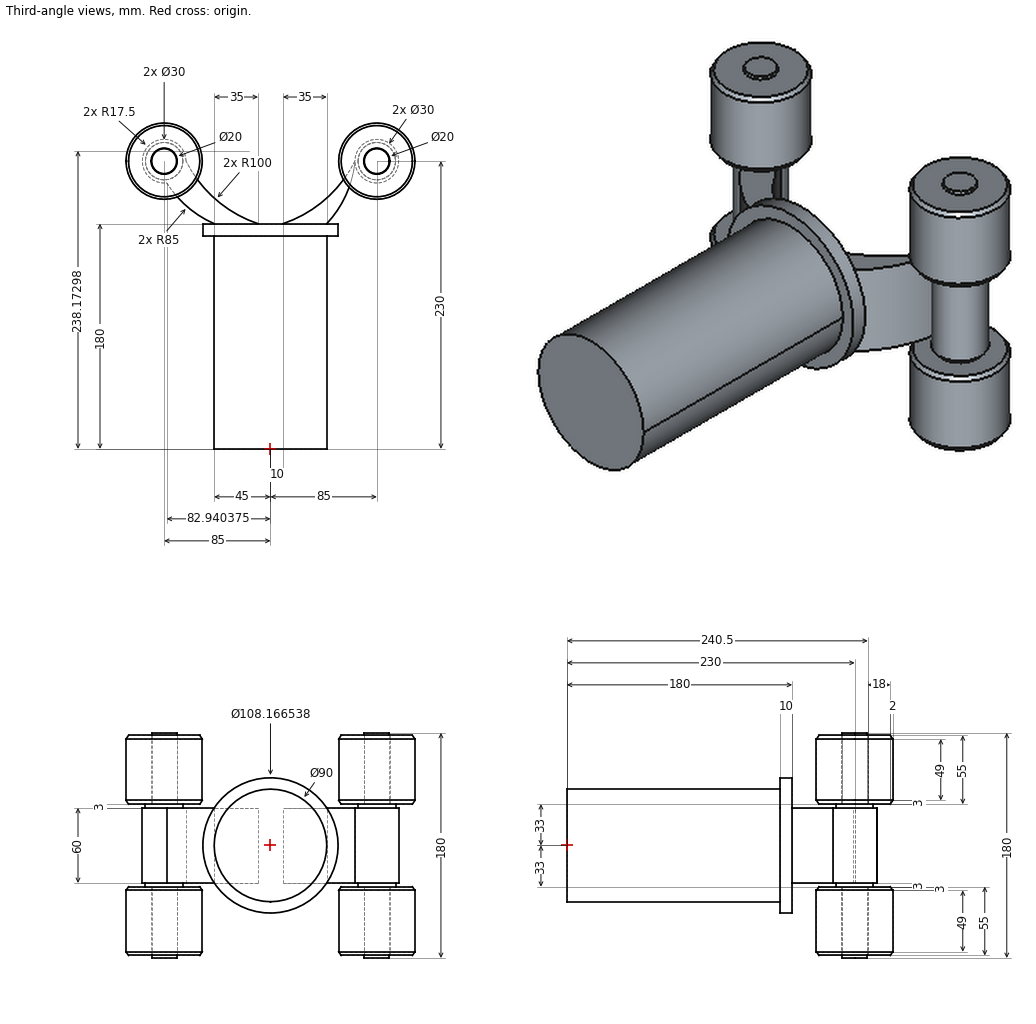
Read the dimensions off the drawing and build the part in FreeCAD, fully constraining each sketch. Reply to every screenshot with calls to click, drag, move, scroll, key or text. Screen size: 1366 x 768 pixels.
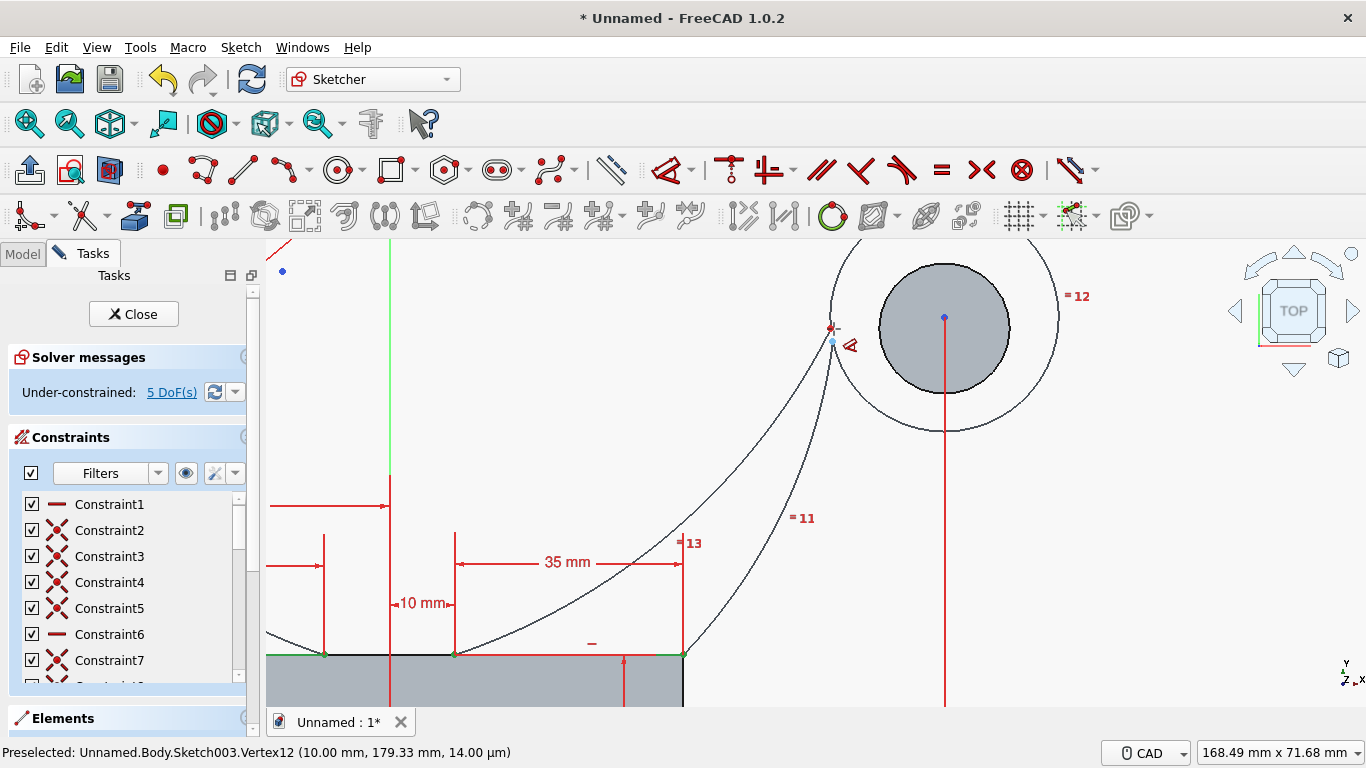
click(831, 329)
click(865, 504)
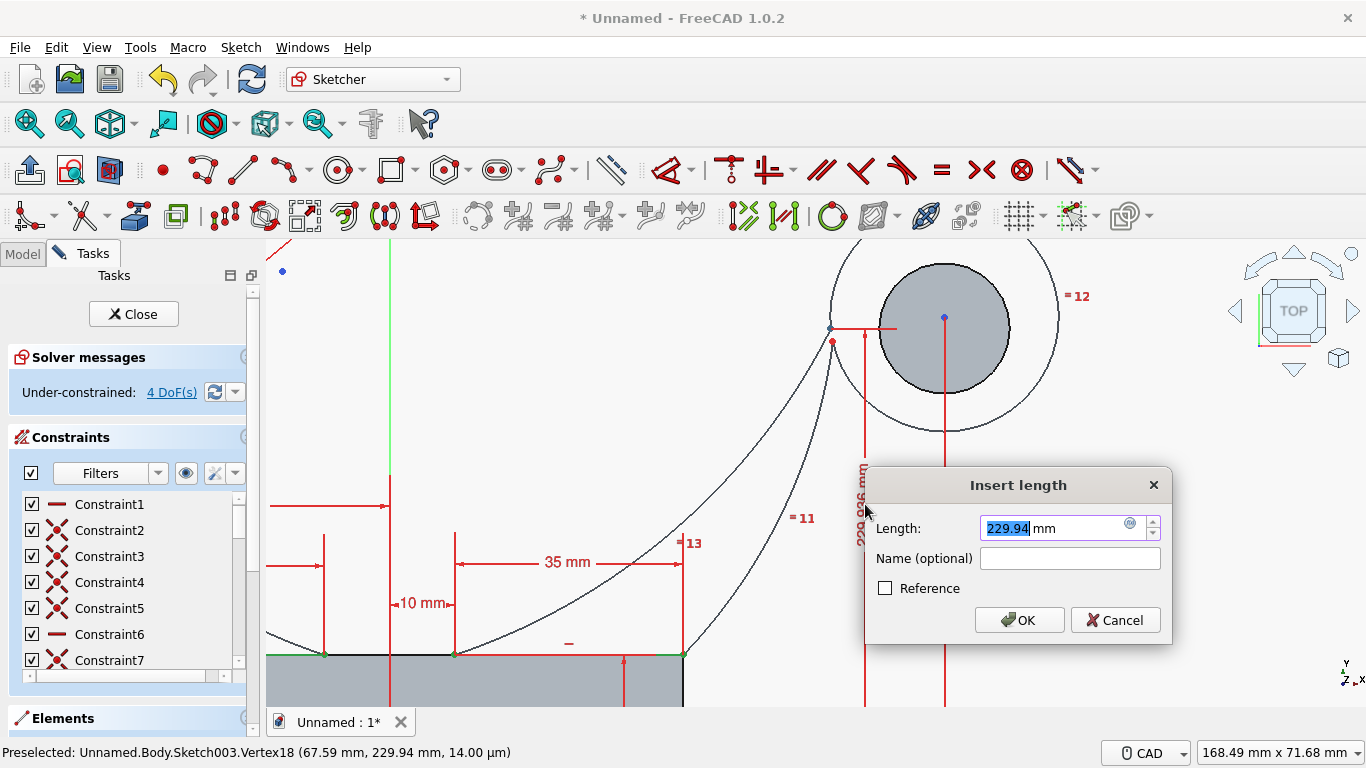
text(230)
key(Return)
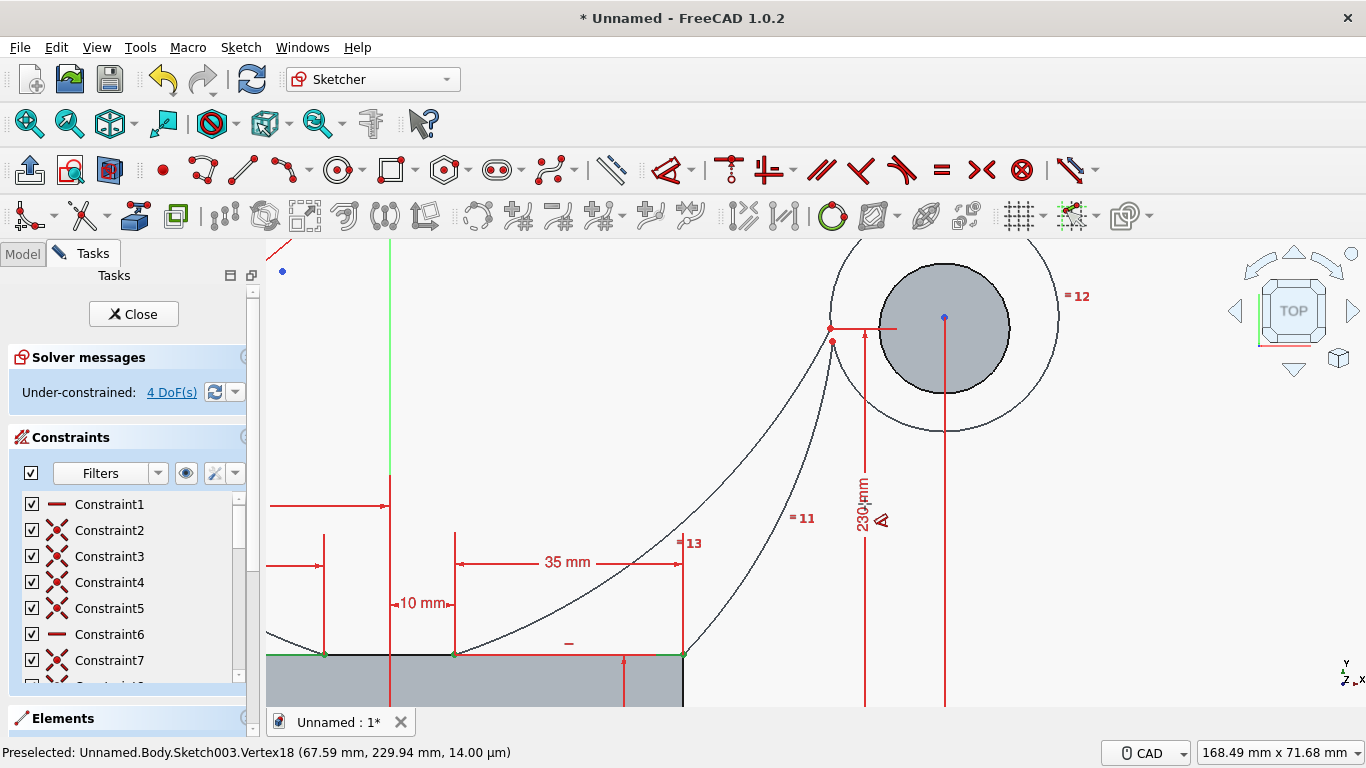
scroll(834, 329, down, 8)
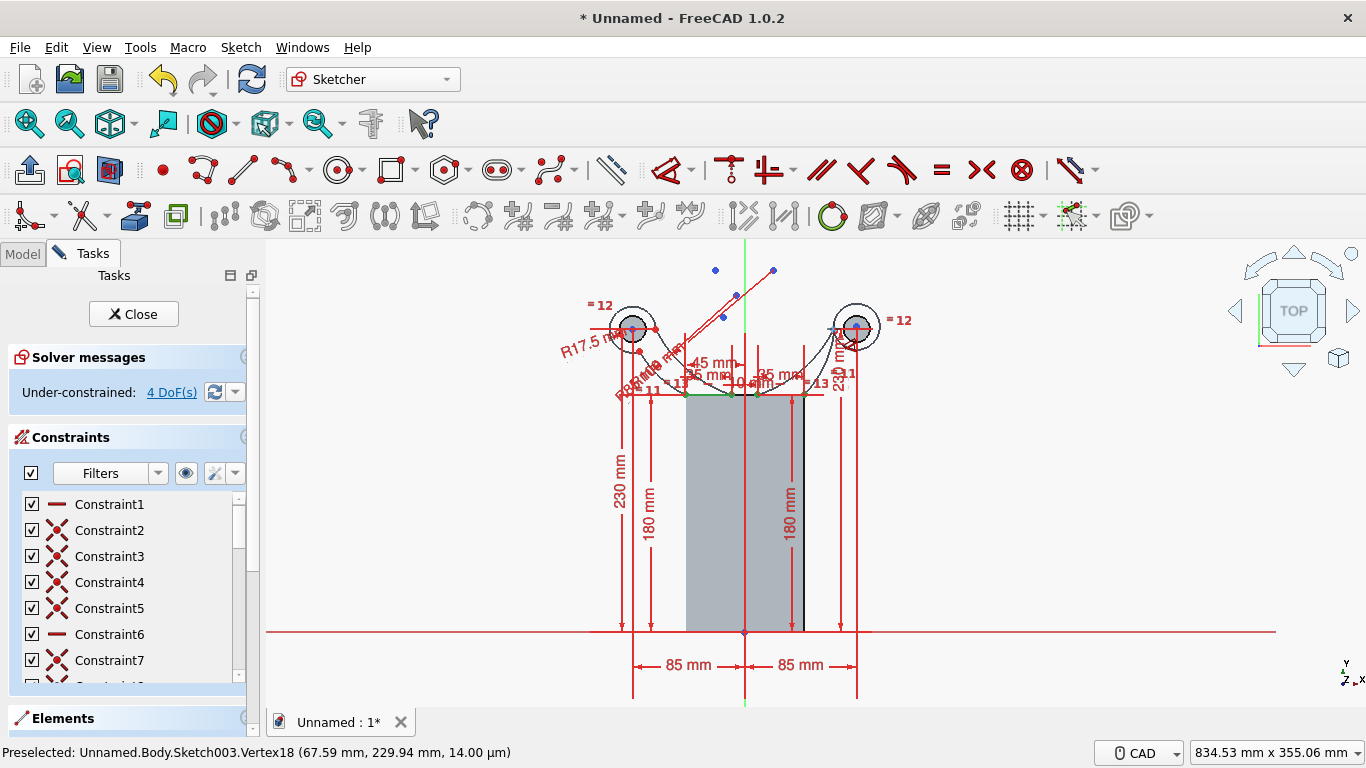
click(633, 330)
click(599, 411)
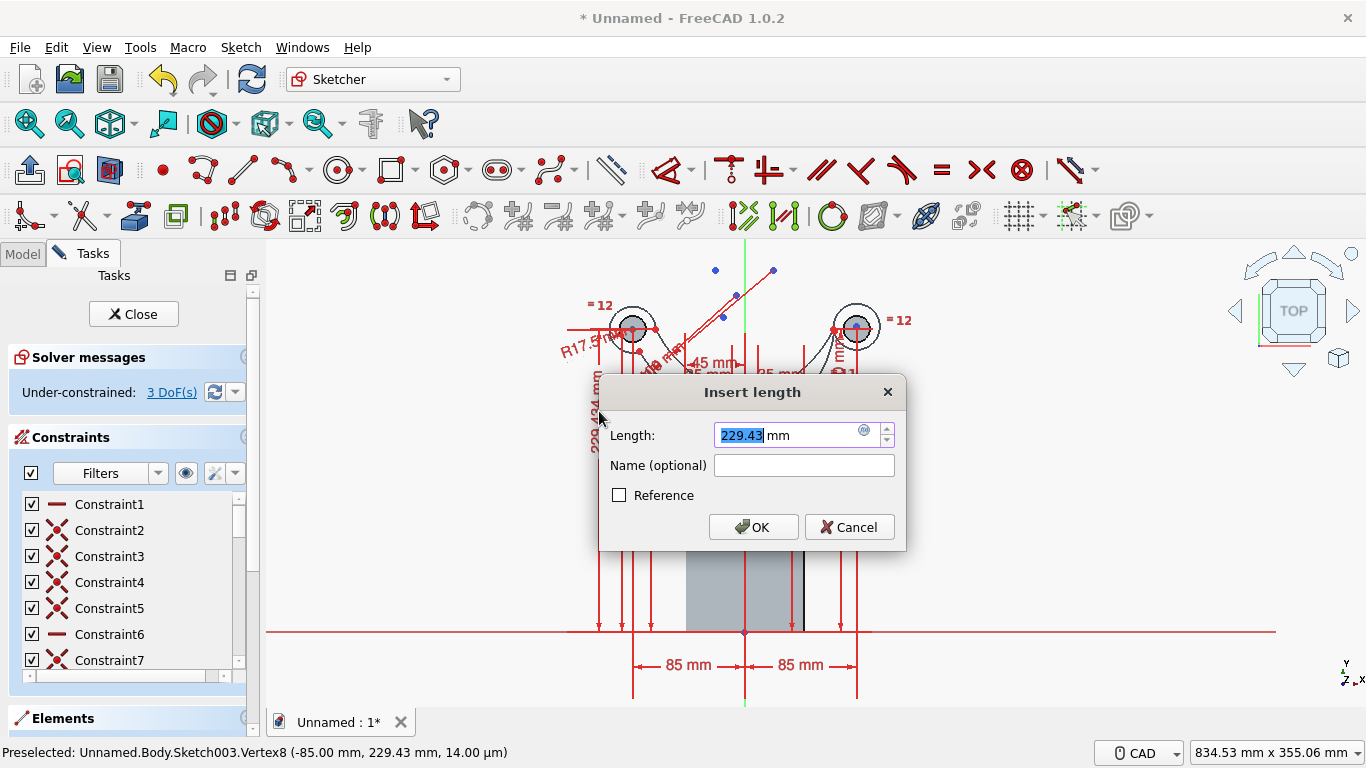
text(230)
key(Return)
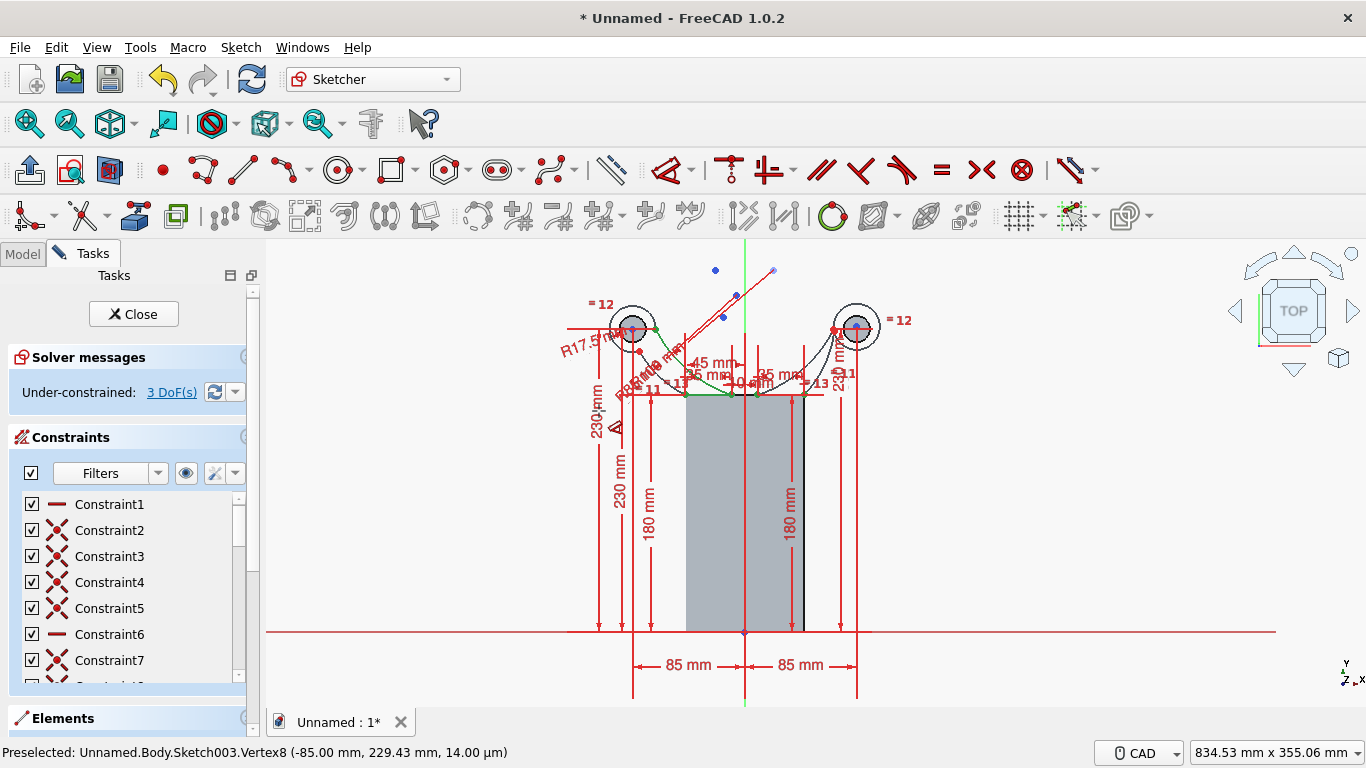
click(857, 327)
click(891, 480)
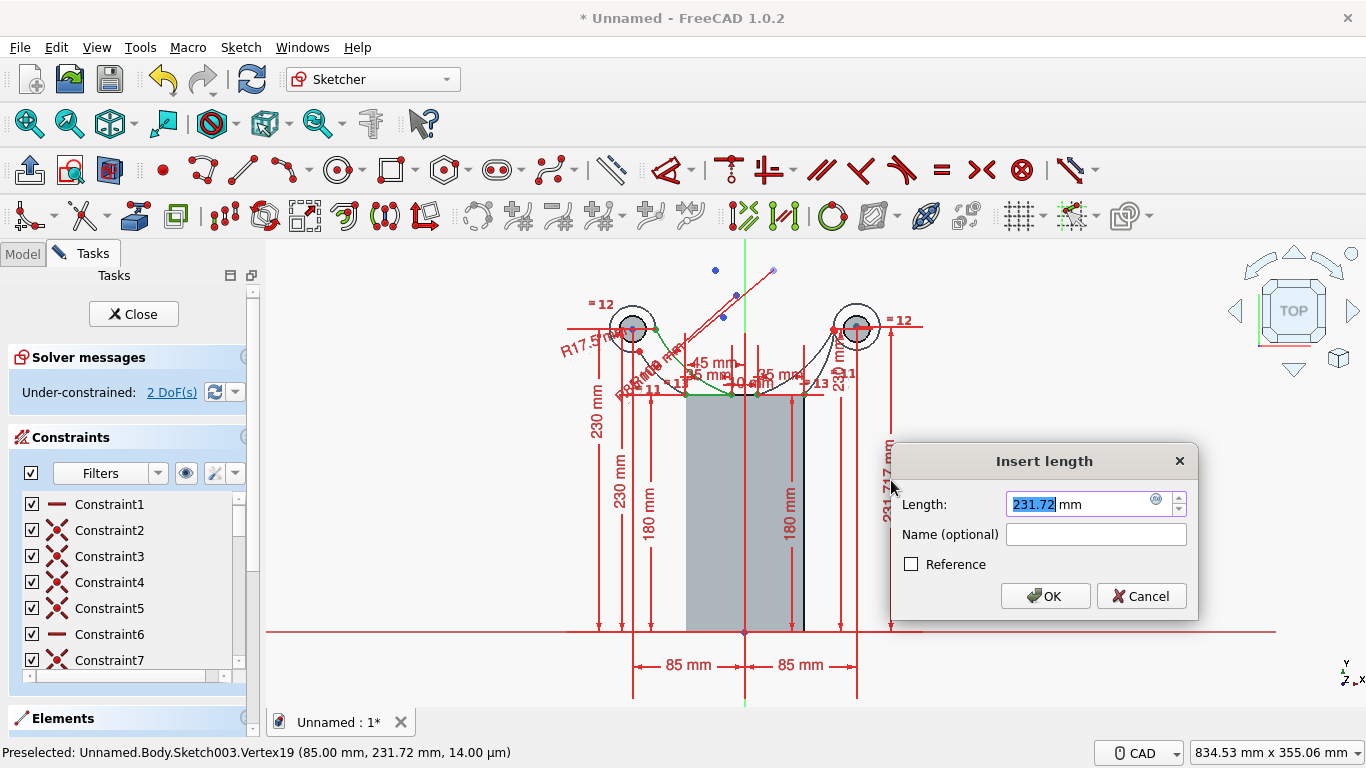
text(230)
key(Return)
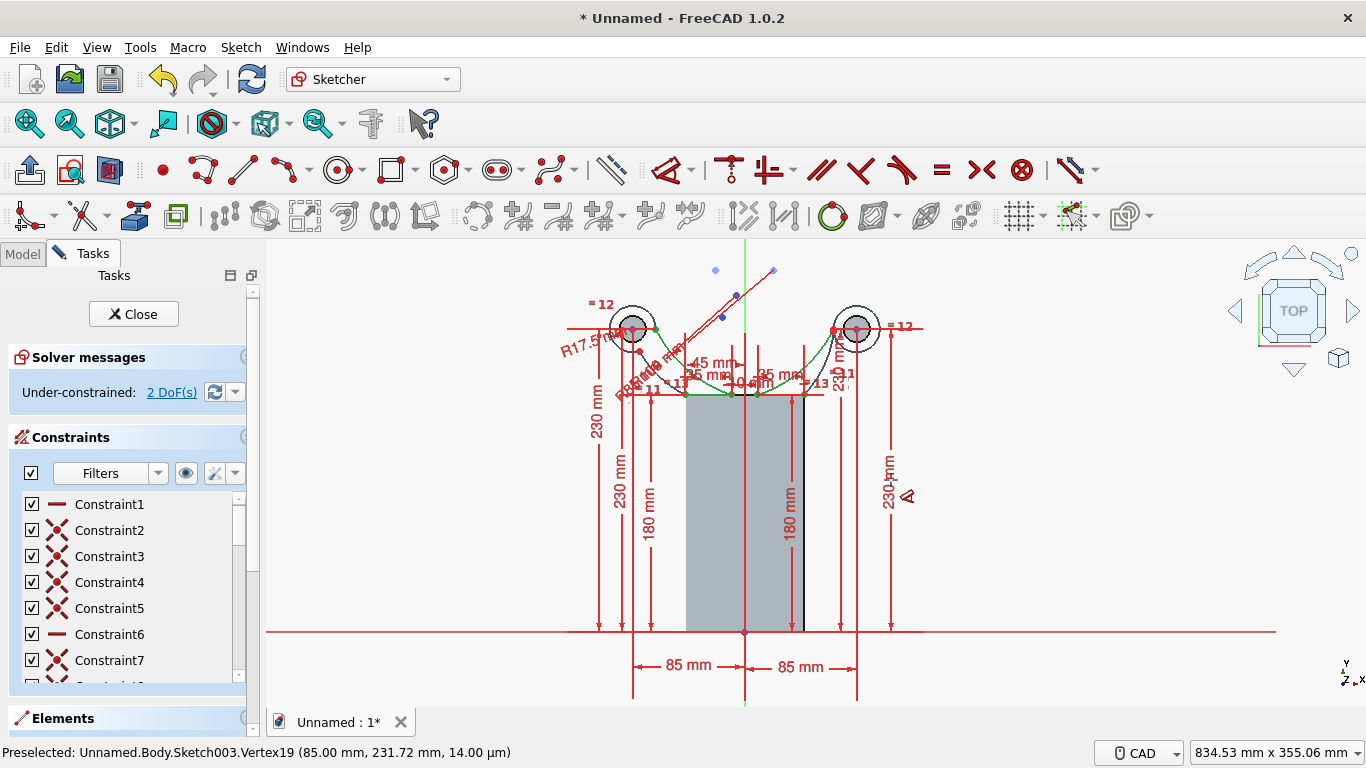
click(639, 351)
click(692, 317)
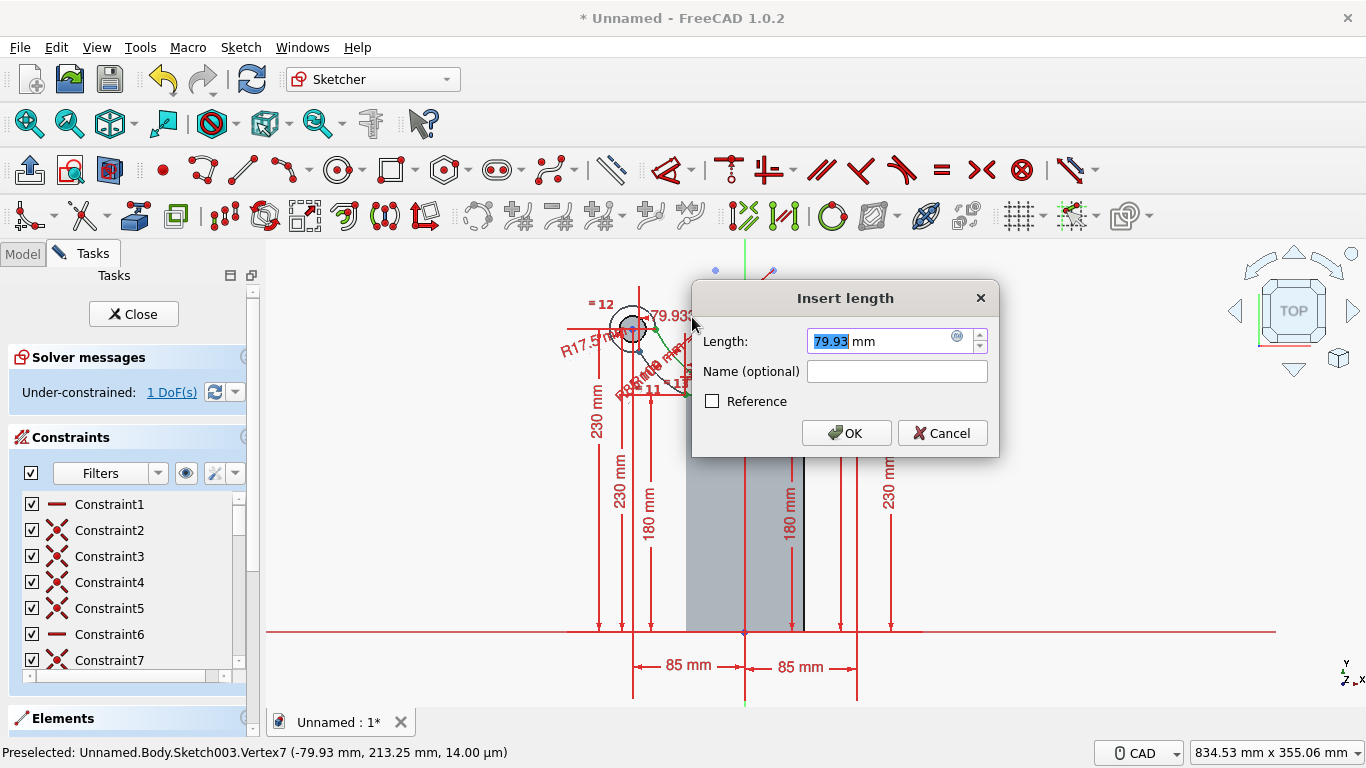
text(82.940375)
key(Return)